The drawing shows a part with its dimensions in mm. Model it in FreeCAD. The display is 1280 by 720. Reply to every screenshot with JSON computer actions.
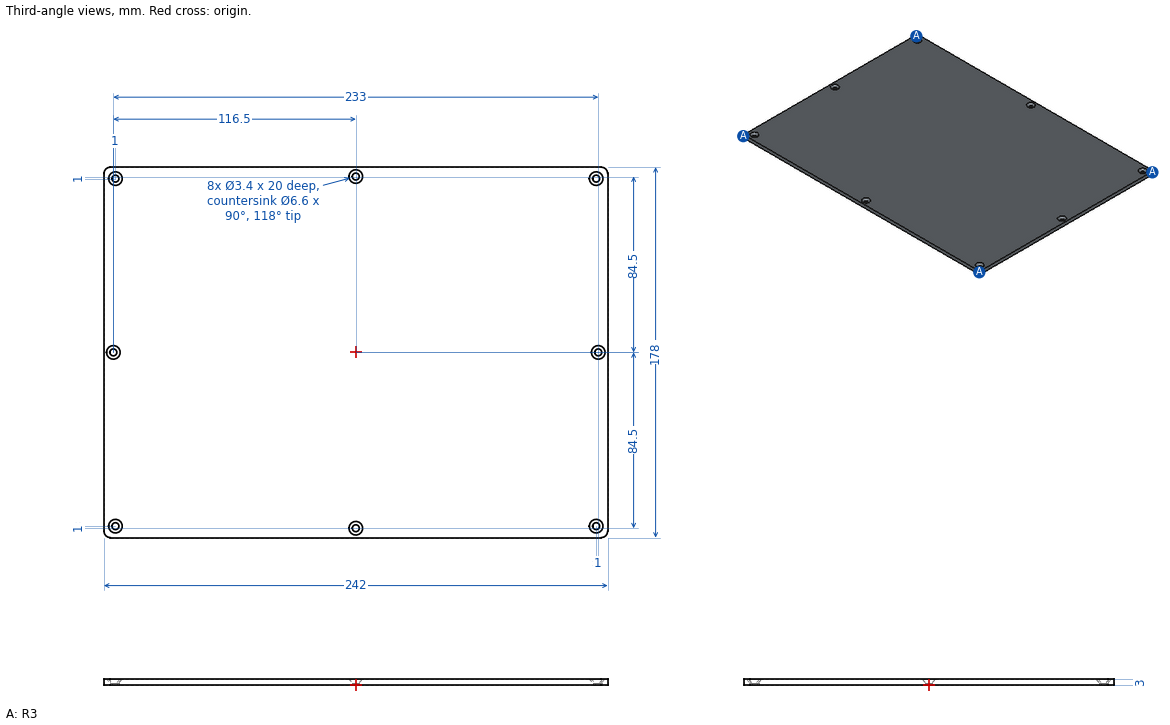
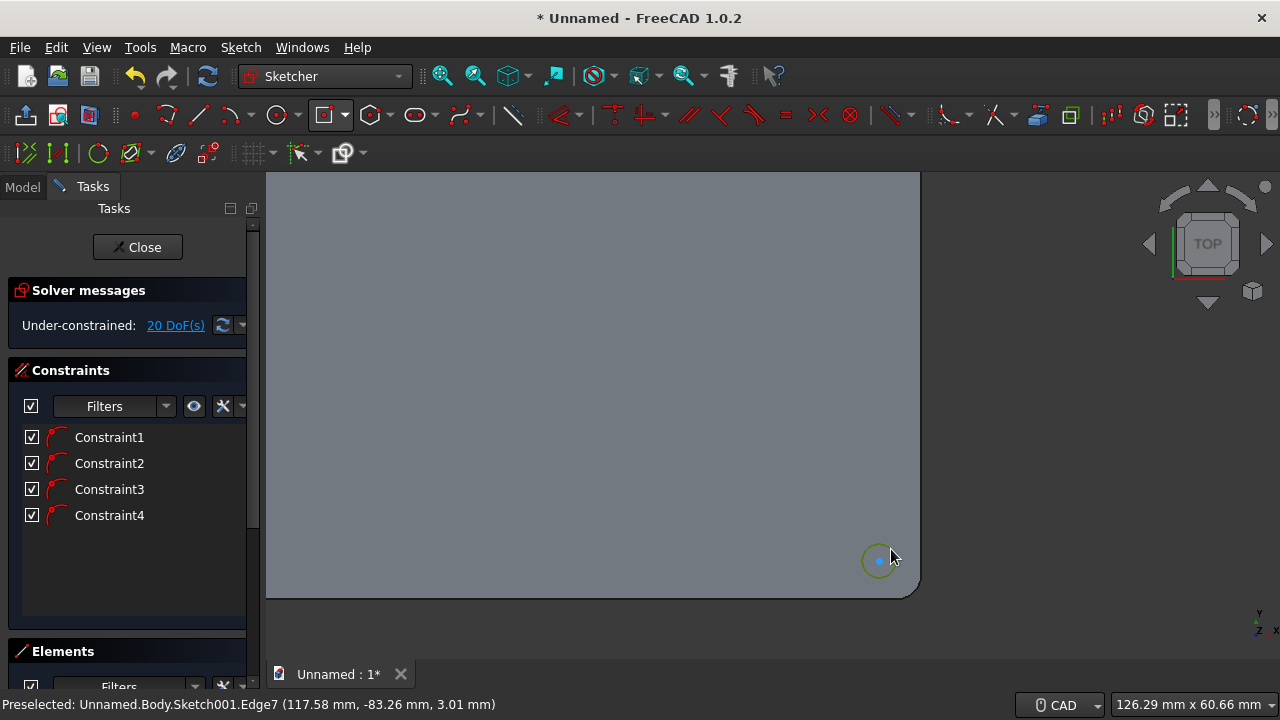
{"action": "scroll", "coordinate": [895, 550], "scroll_direction": "down", "scroll_amount": 8}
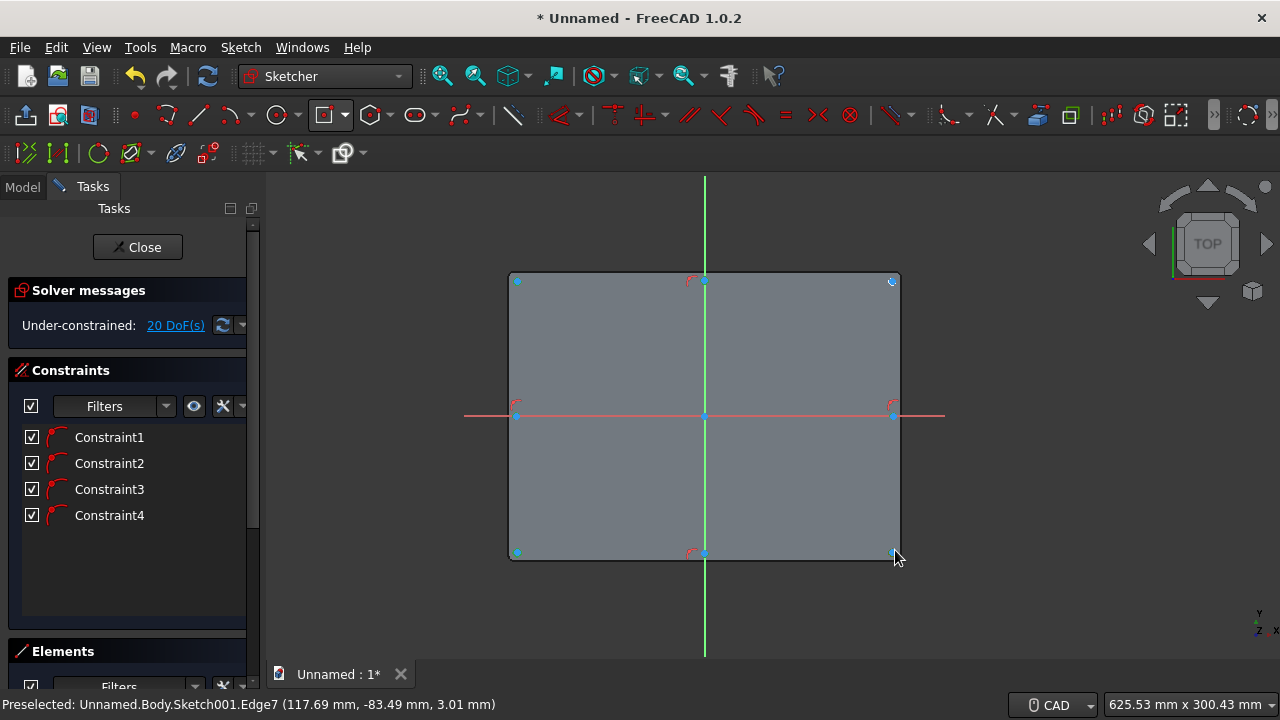
{"action": "scroll", "coordinate": [894, 280], "scroll_direction": "up", "scroll_amount": 8}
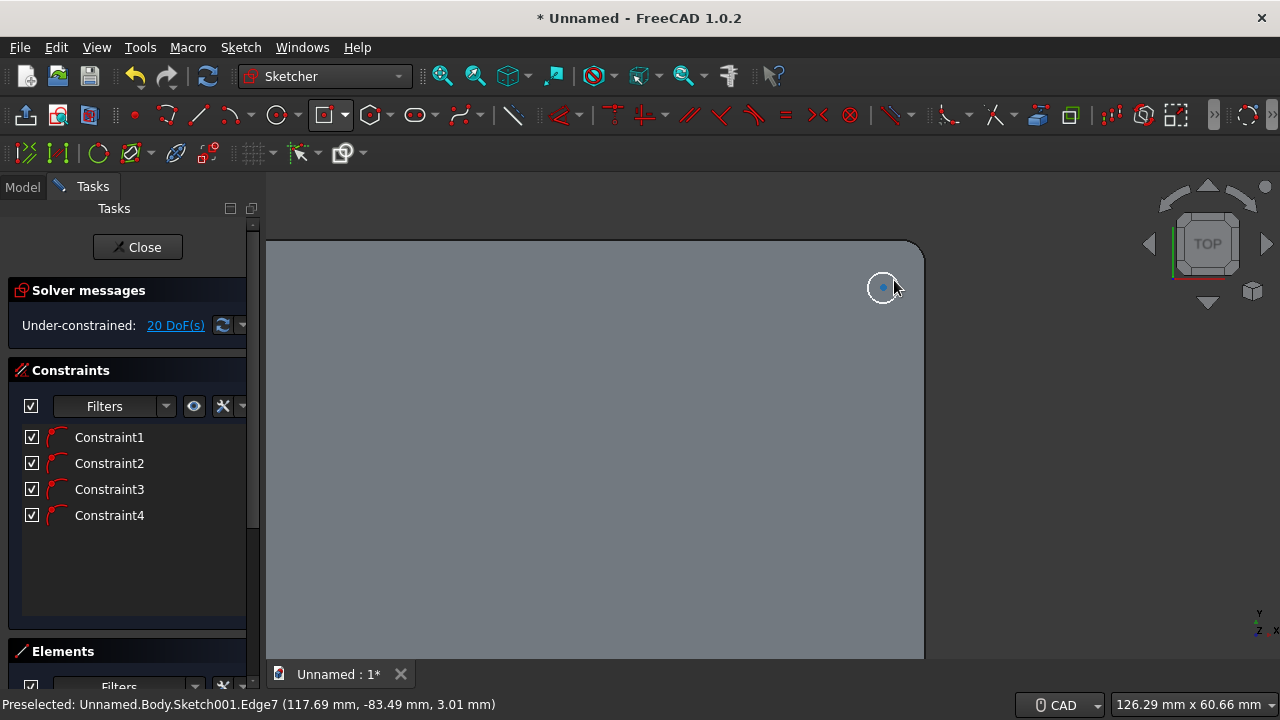
{"action": "left_click", "coordinate": [894, 277]}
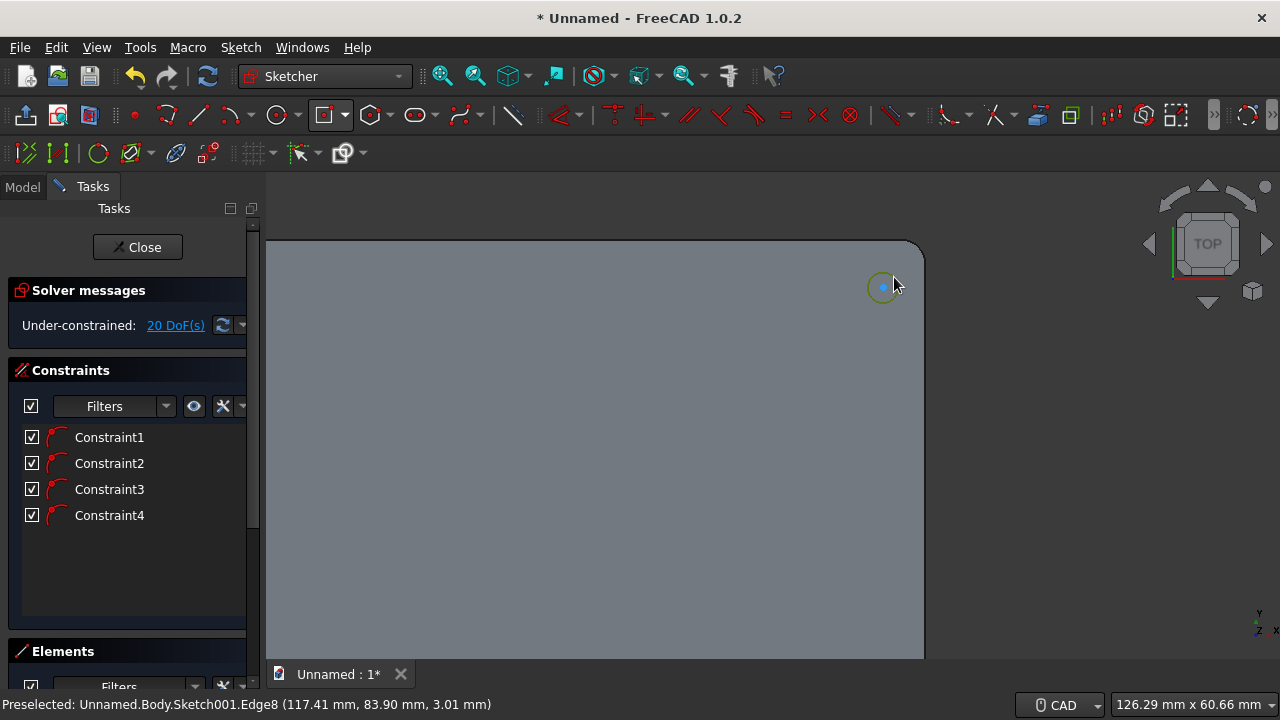
{"action": "left_click", "coordinate": [786, 116]}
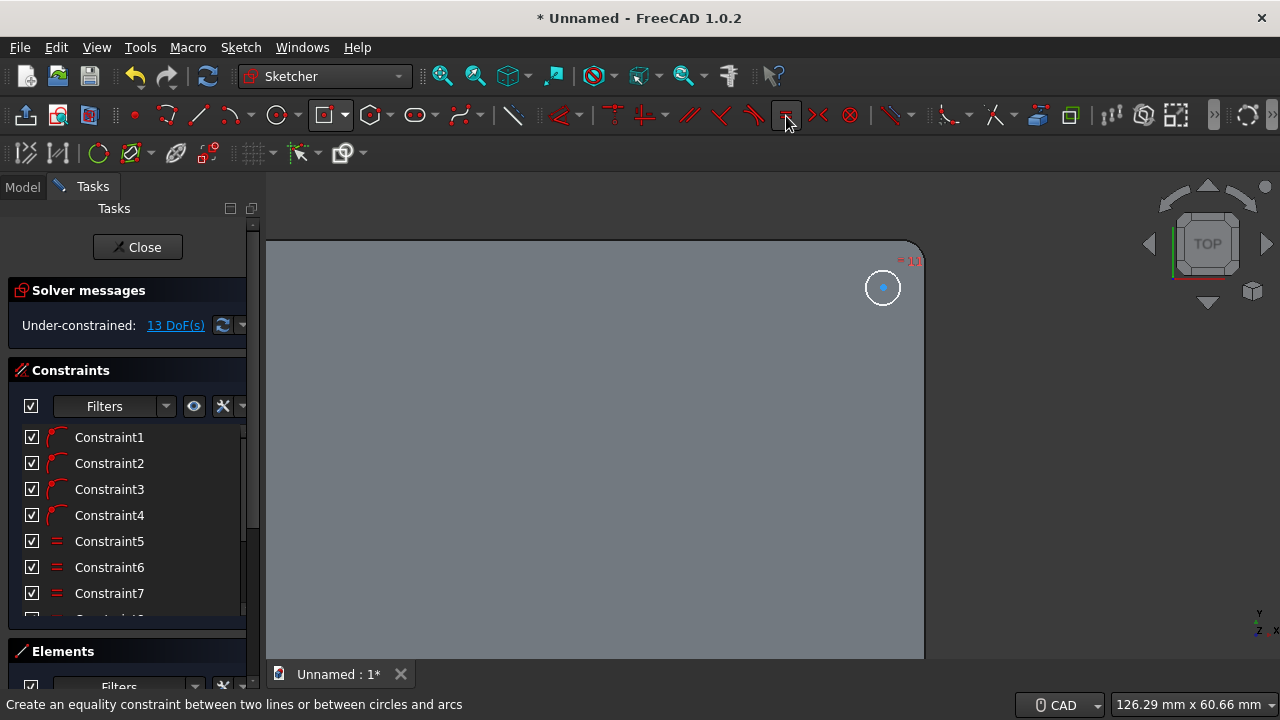
{"action": "scroll", "coordinate": [894, 279], "scroll_direction": "down", "scroll_amount": 8}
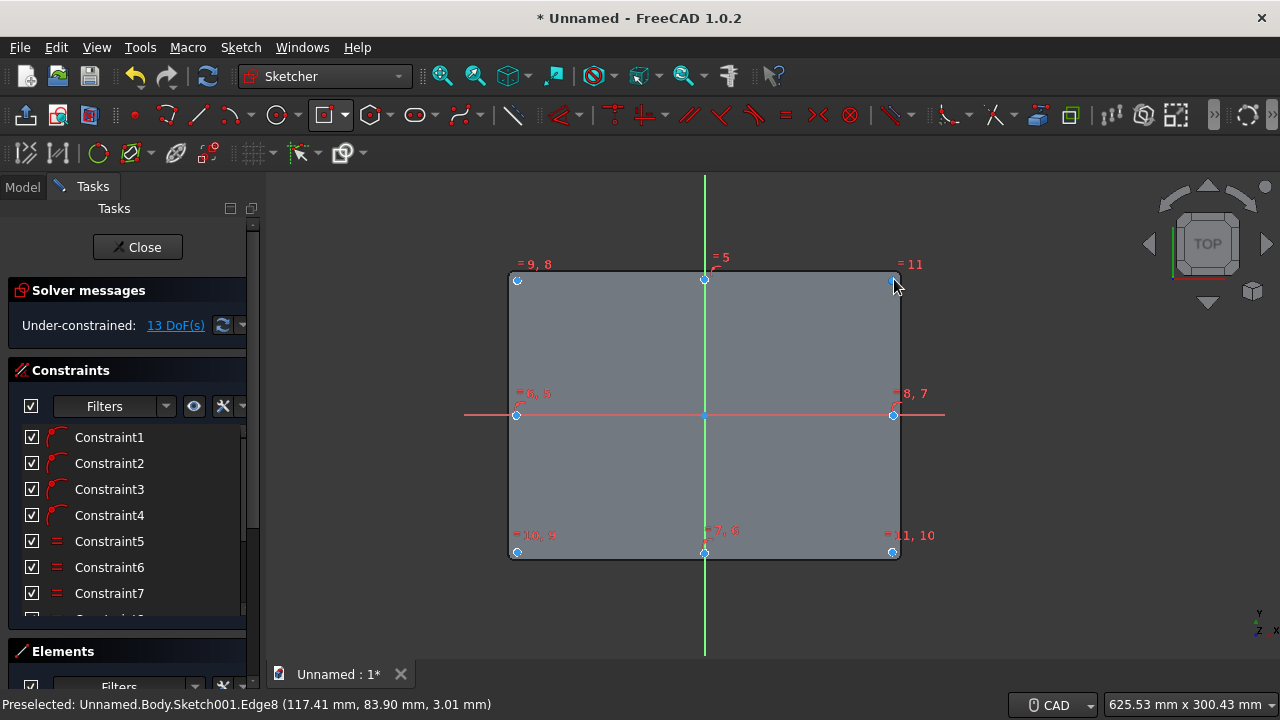
{"action": "left_click", "coordinate": [517, 281]}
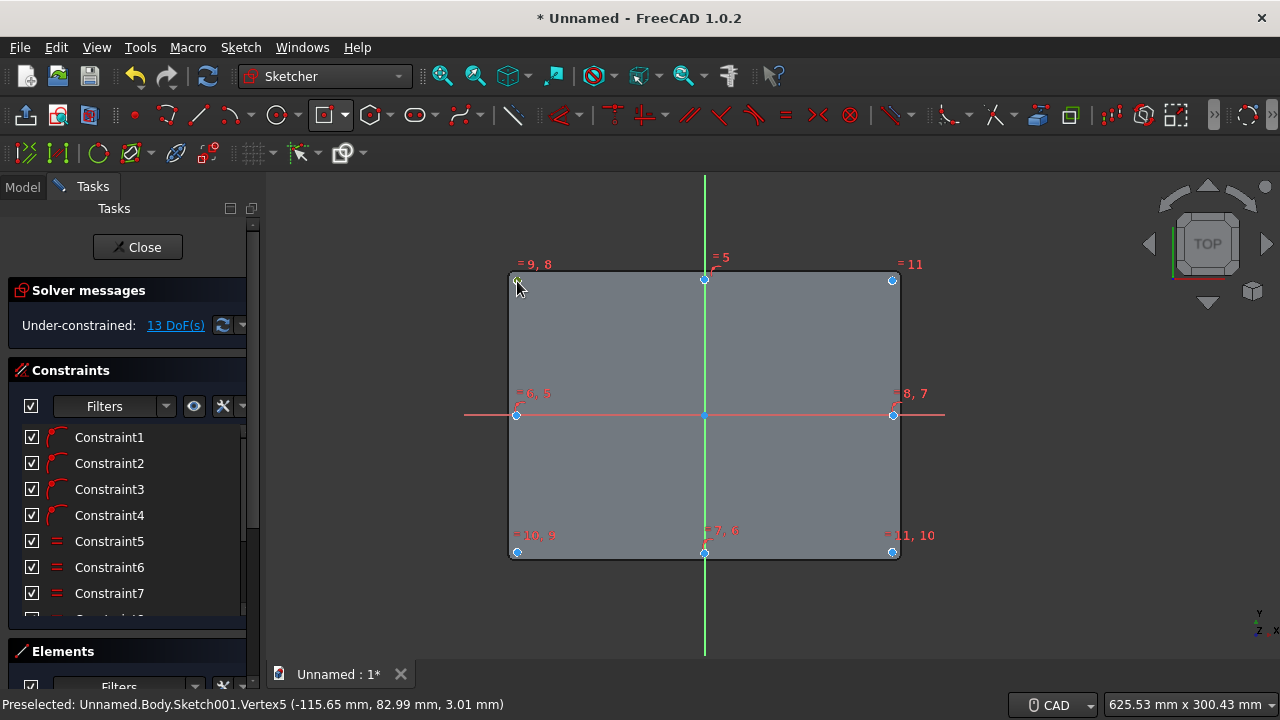
{"action": "left_click", "coordinate": [517, 552]}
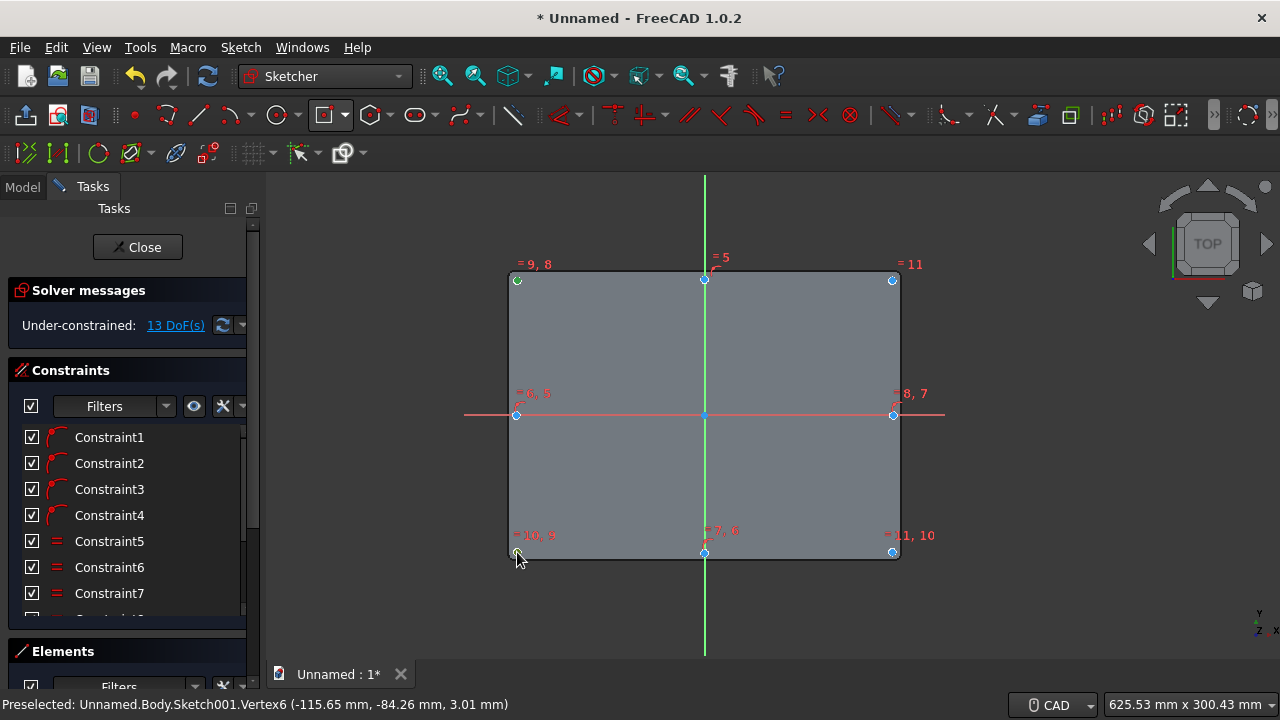
{"action": "left_click", "coordinate": [668, 116]}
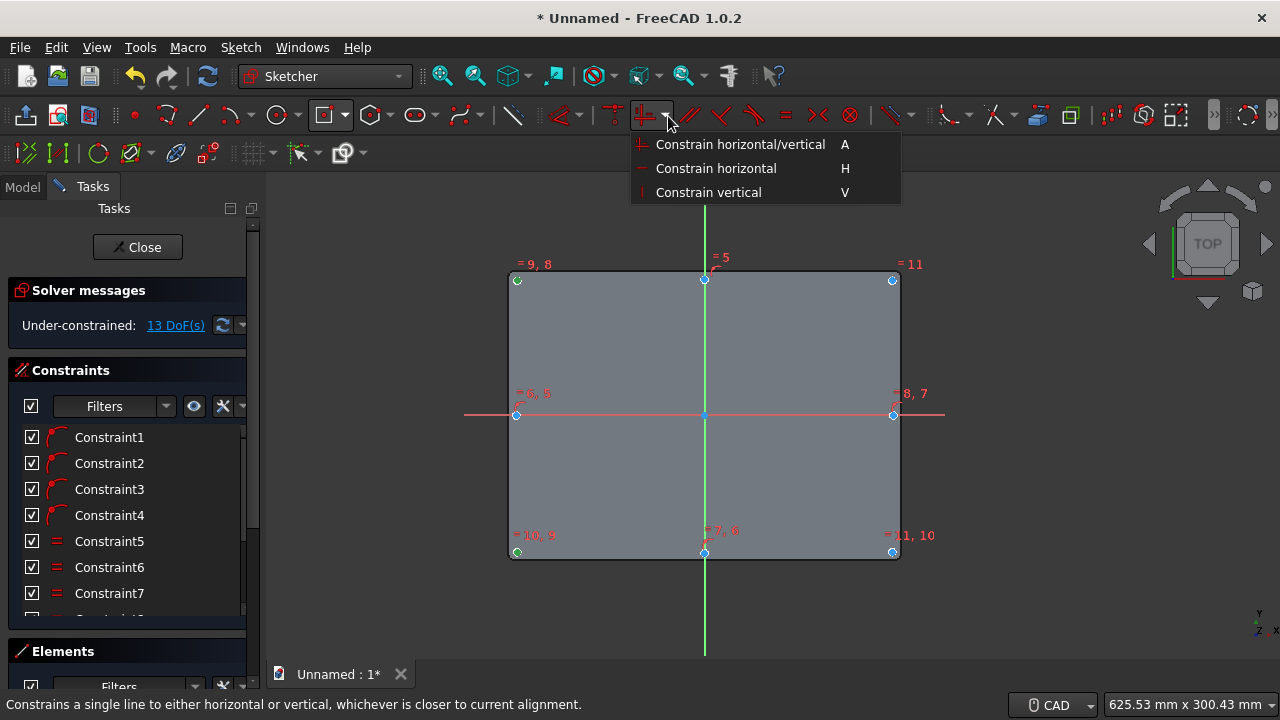
{"action": "left_click", "coordinate": [766, 192]}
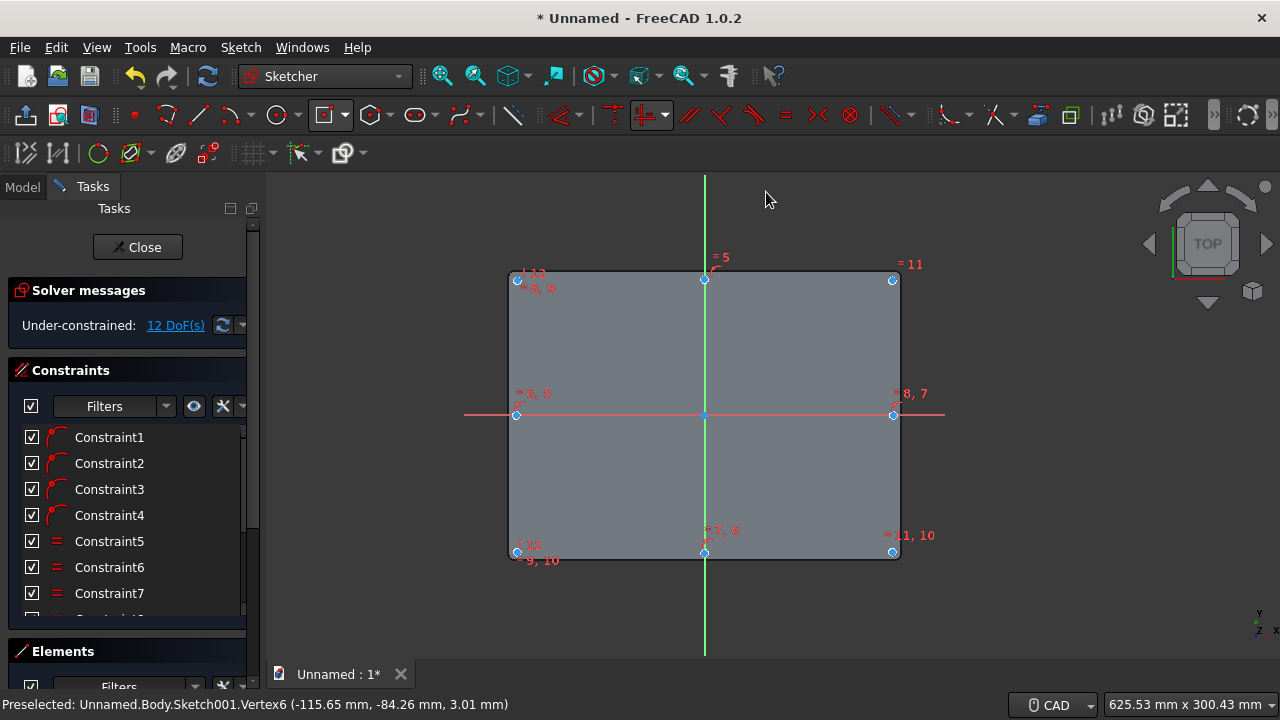
{"action": "scroll", "coordinate": [517, 552], "scroll_direction": "up", "scroll_amount": 4}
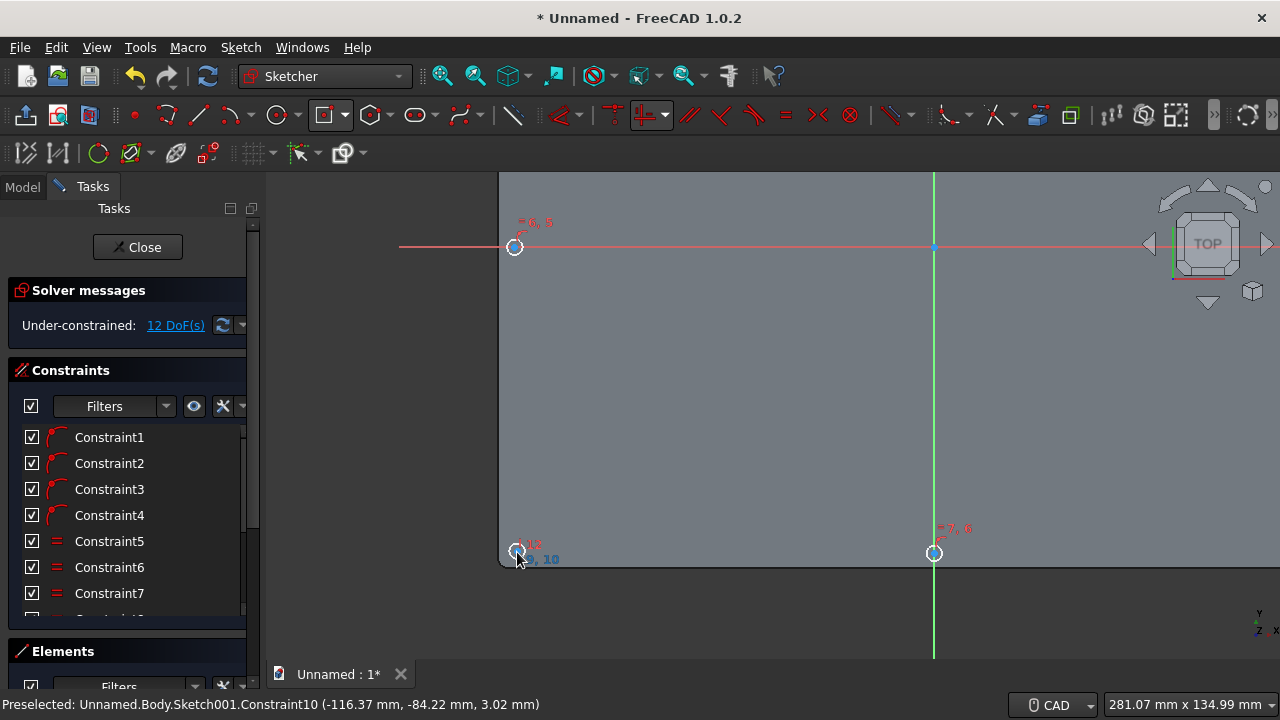
{"action": "scroll", "coordinate": [517, 551], "scroll_direction": "up", "scroll_amount": 4}